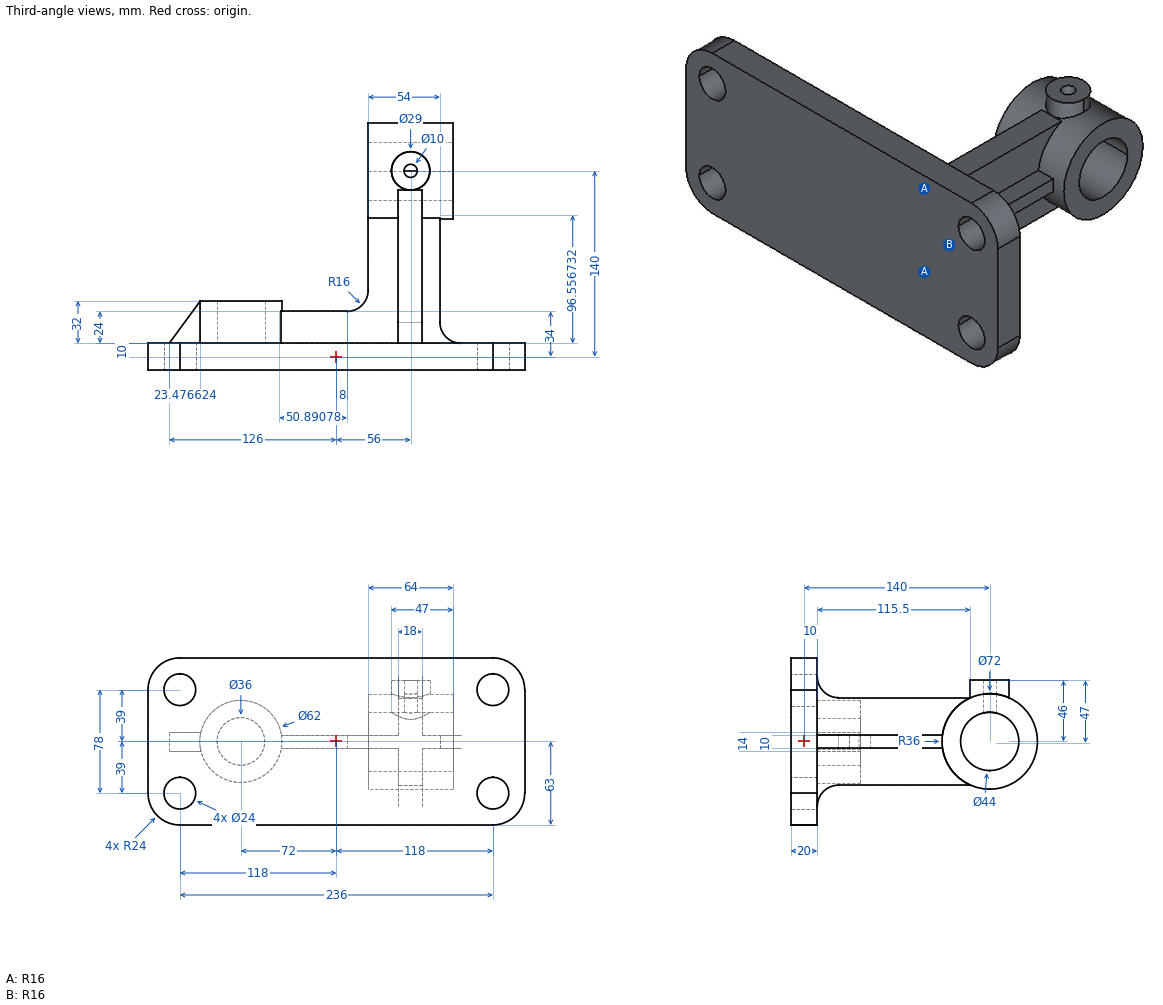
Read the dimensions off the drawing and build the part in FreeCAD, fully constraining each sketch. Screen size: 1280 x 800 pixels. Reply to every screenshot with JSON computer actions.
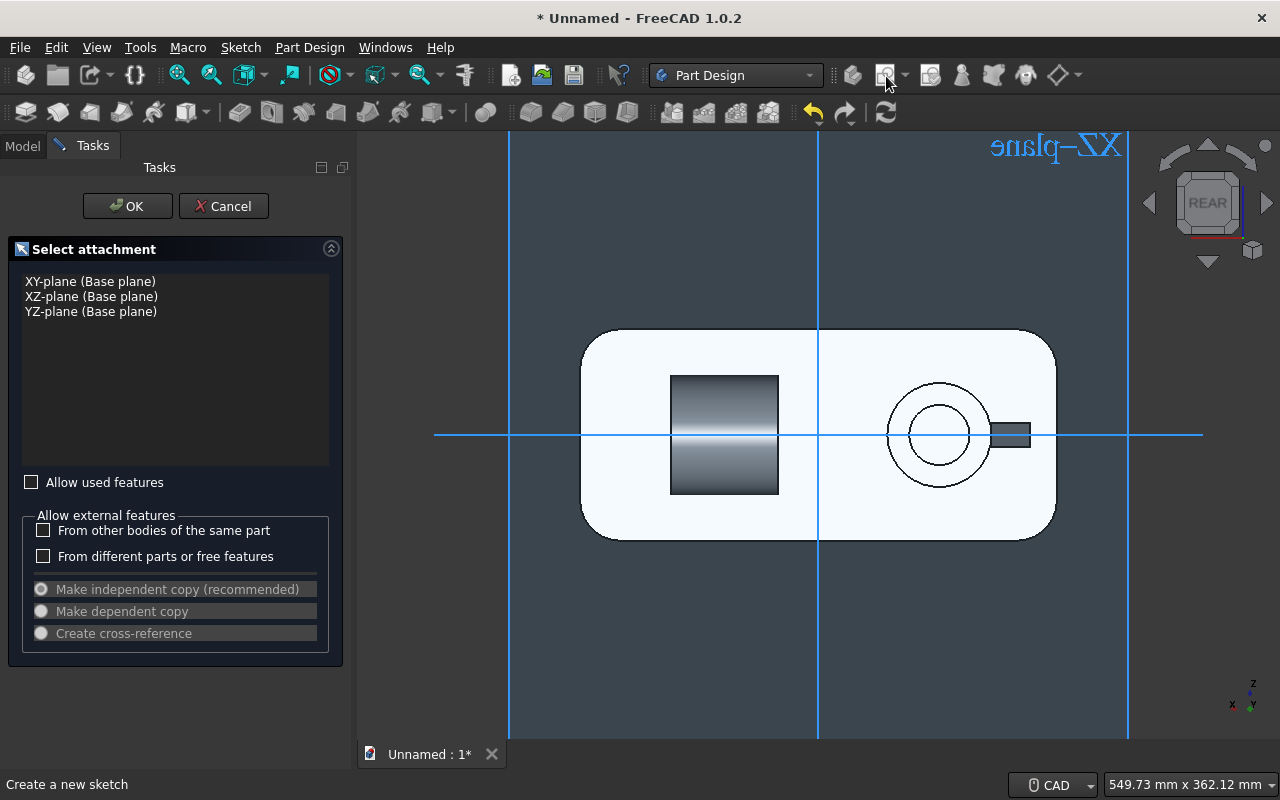
{"action": "left_click", "coordinate": [82, 282]}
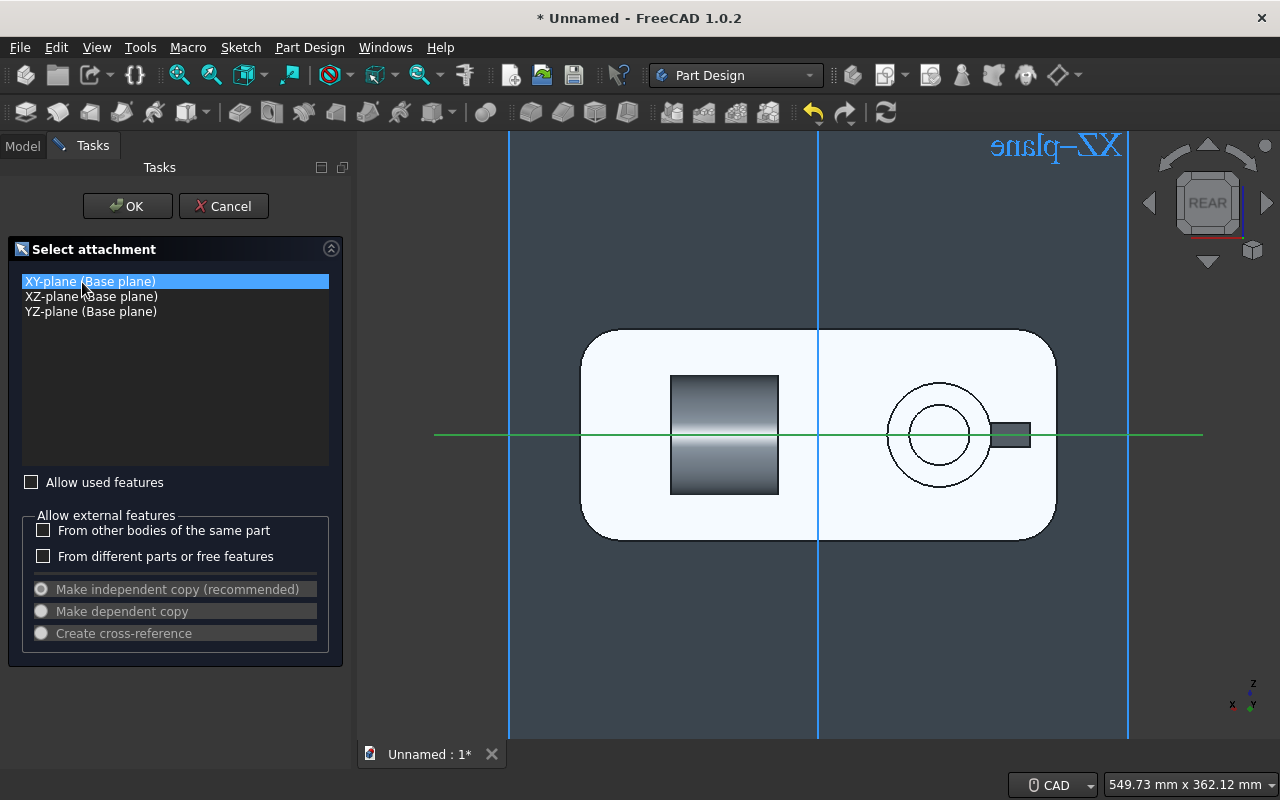
{"action": "left_click", "coordinate": [128, 206]}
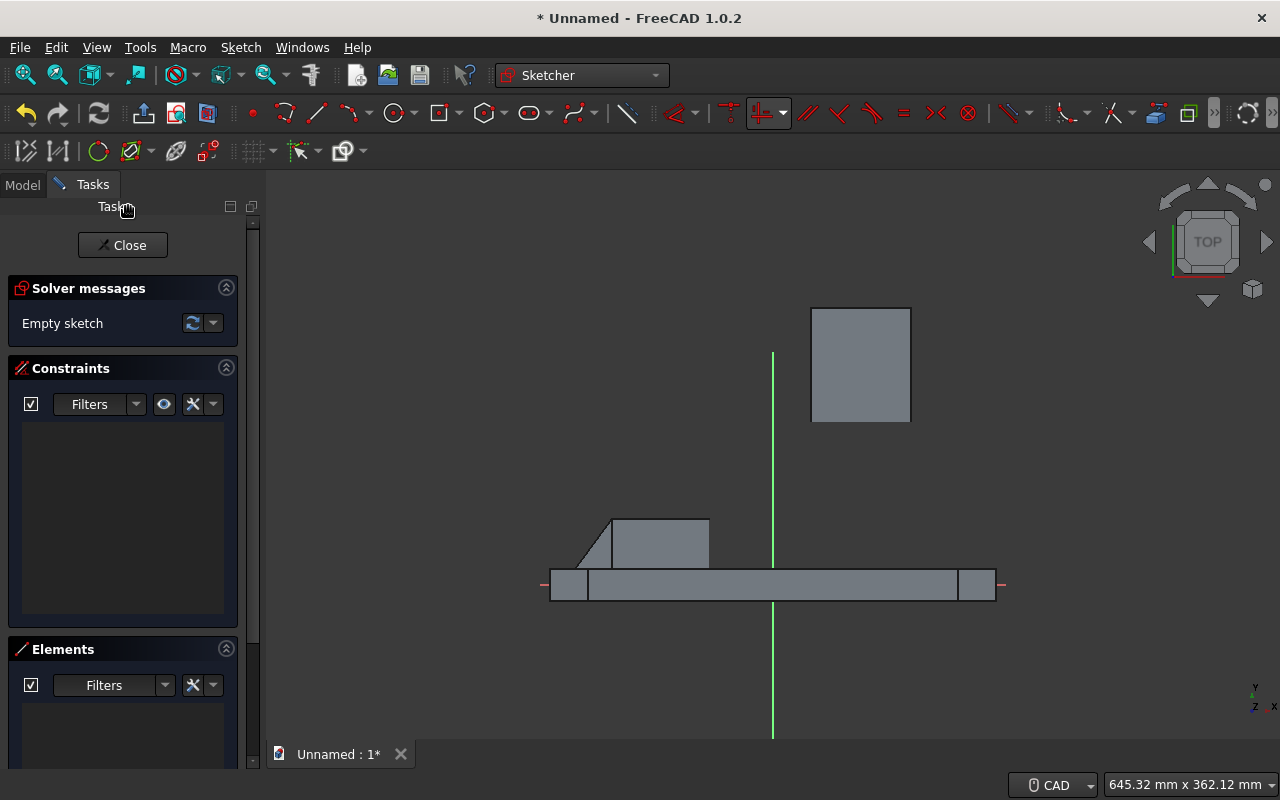
{"action": "left_click", "coordinate": [208, 114]}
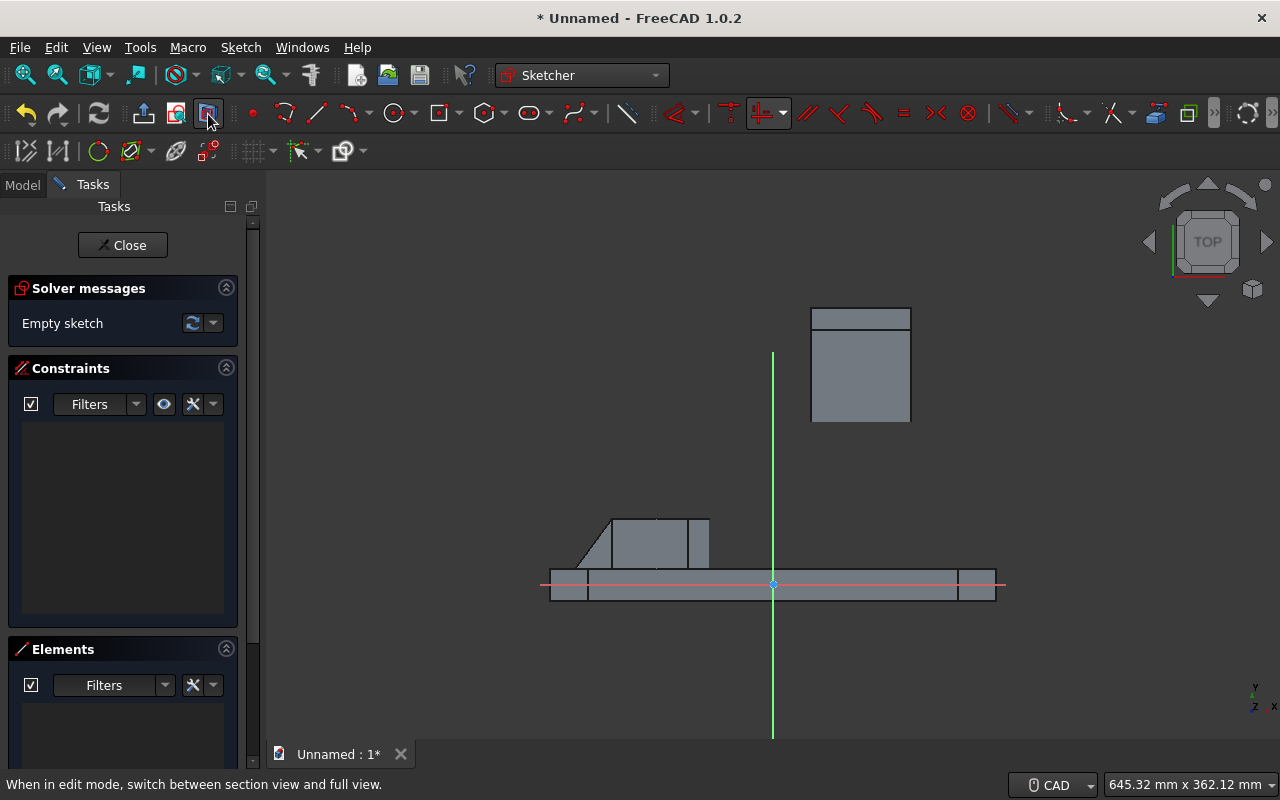
{"action": "scroll", "coordinate": [879, 539], "scroll_direction": "up", "scroll_amount": 4}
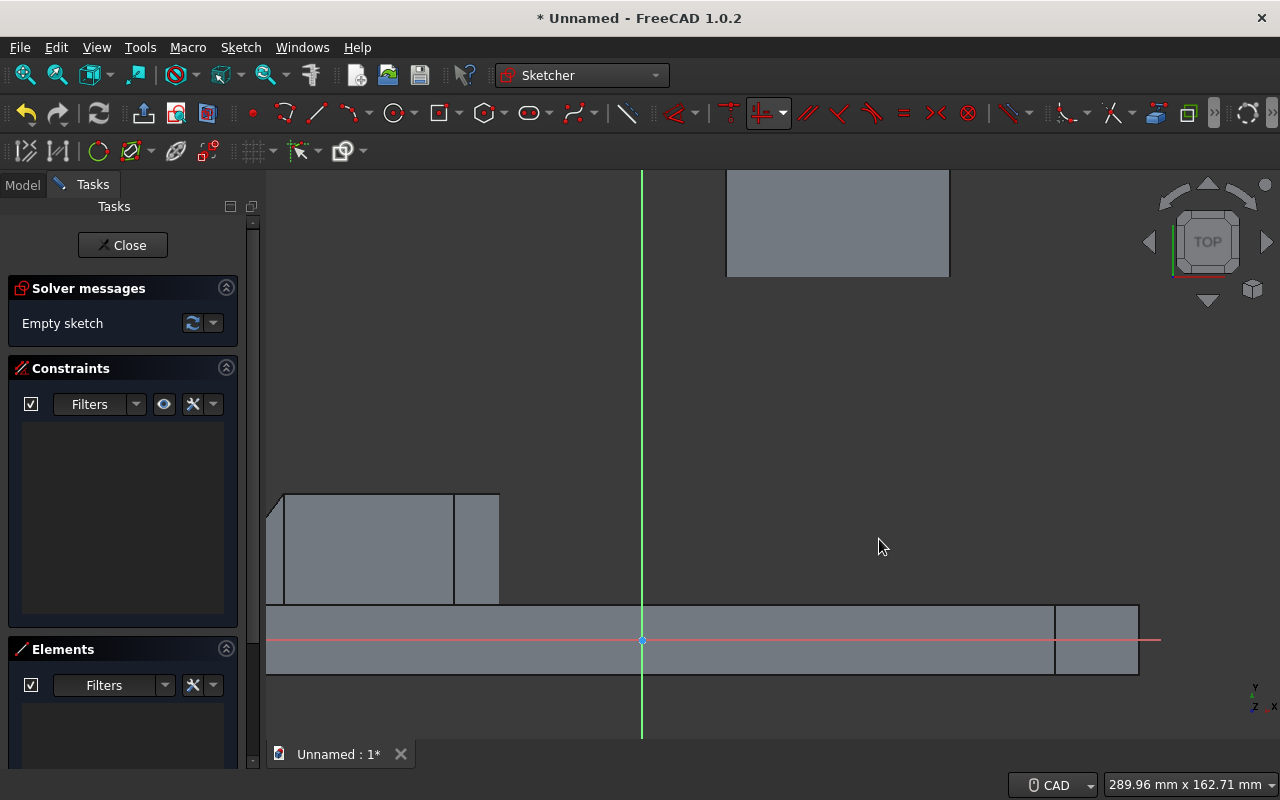
{"action": "left_click", "coordinate": [286, 114]}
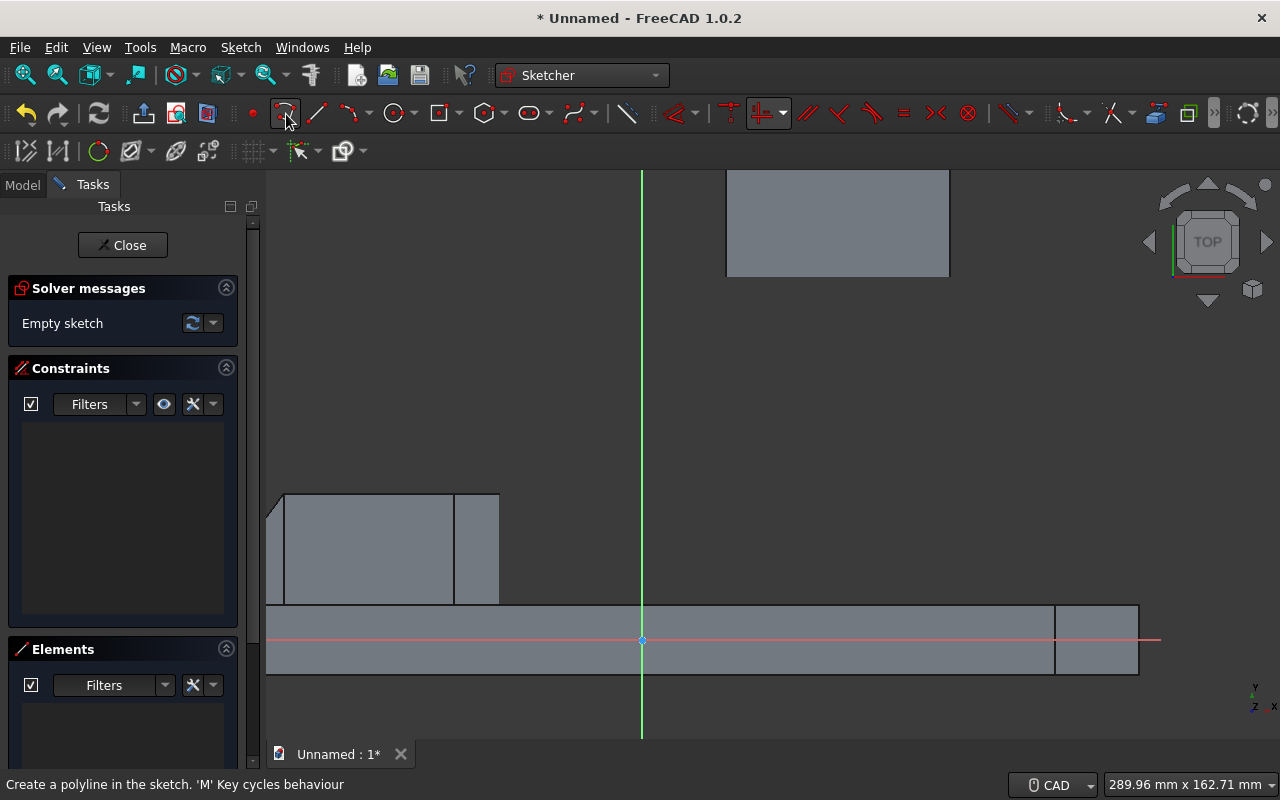
{"action": "left_click", "coordinate": [670, 522]}
{"action": "left_click", "coordinate": [492, 522]}
{"action": "left_click", "coordinate": [492, 605]}
{"action": "left_click", "coordinate": [915, 605]}
{"action": "left_click", "coordinate": [915, 268]}
{"action": "left_click", "coordinate": [726, 268]}
{"action": "left_click", "coordinate": [726, 466]}
{"action": "right_click", "coordinate": [726, 466]}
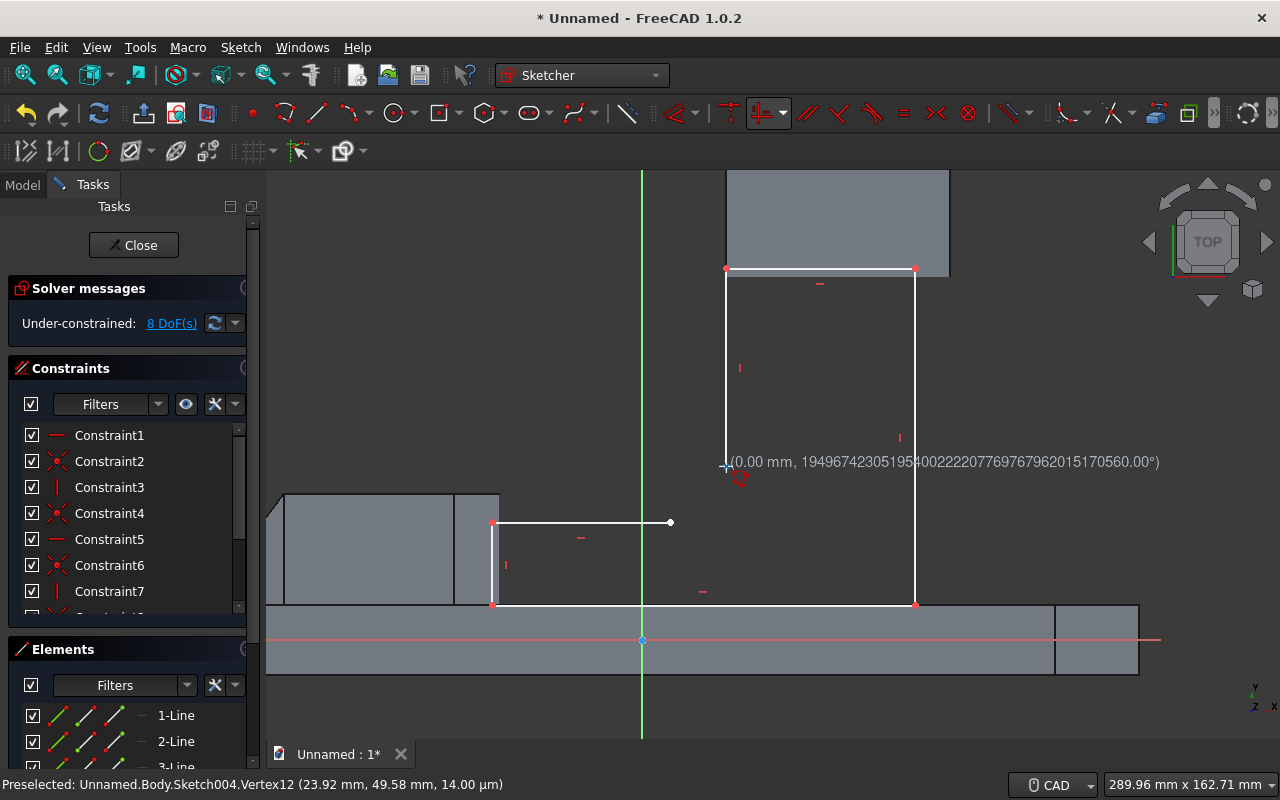
{"action": "left_click", "coordinate": [350, 114]}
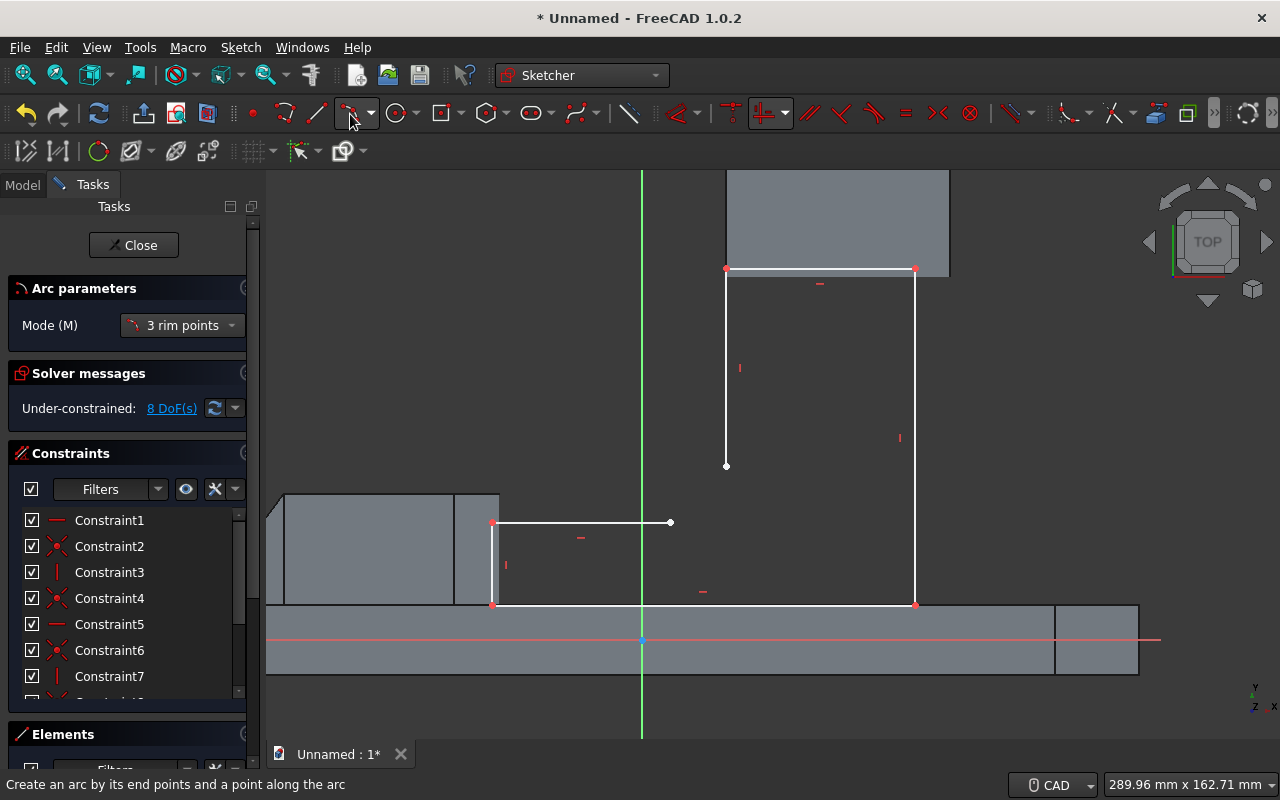
{"action": "left_click", "coordinate": [726, 467]}
{"action": "left_click", "coordinate": [670, 523]}
{"action": "left_click", "coordinate": [710, 505]}
{"action": "key", "text": "Escape"}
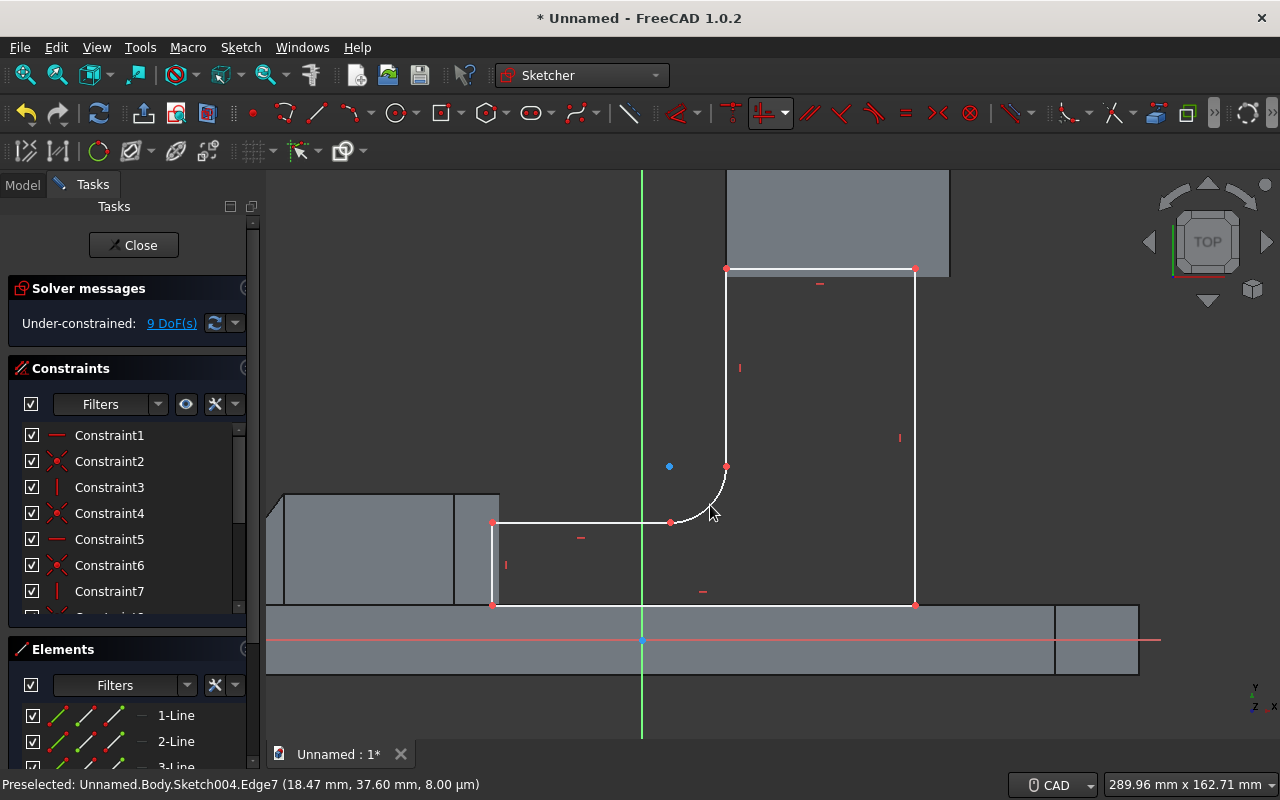
{"action": "left_click", "coordinate": [617, 523]}